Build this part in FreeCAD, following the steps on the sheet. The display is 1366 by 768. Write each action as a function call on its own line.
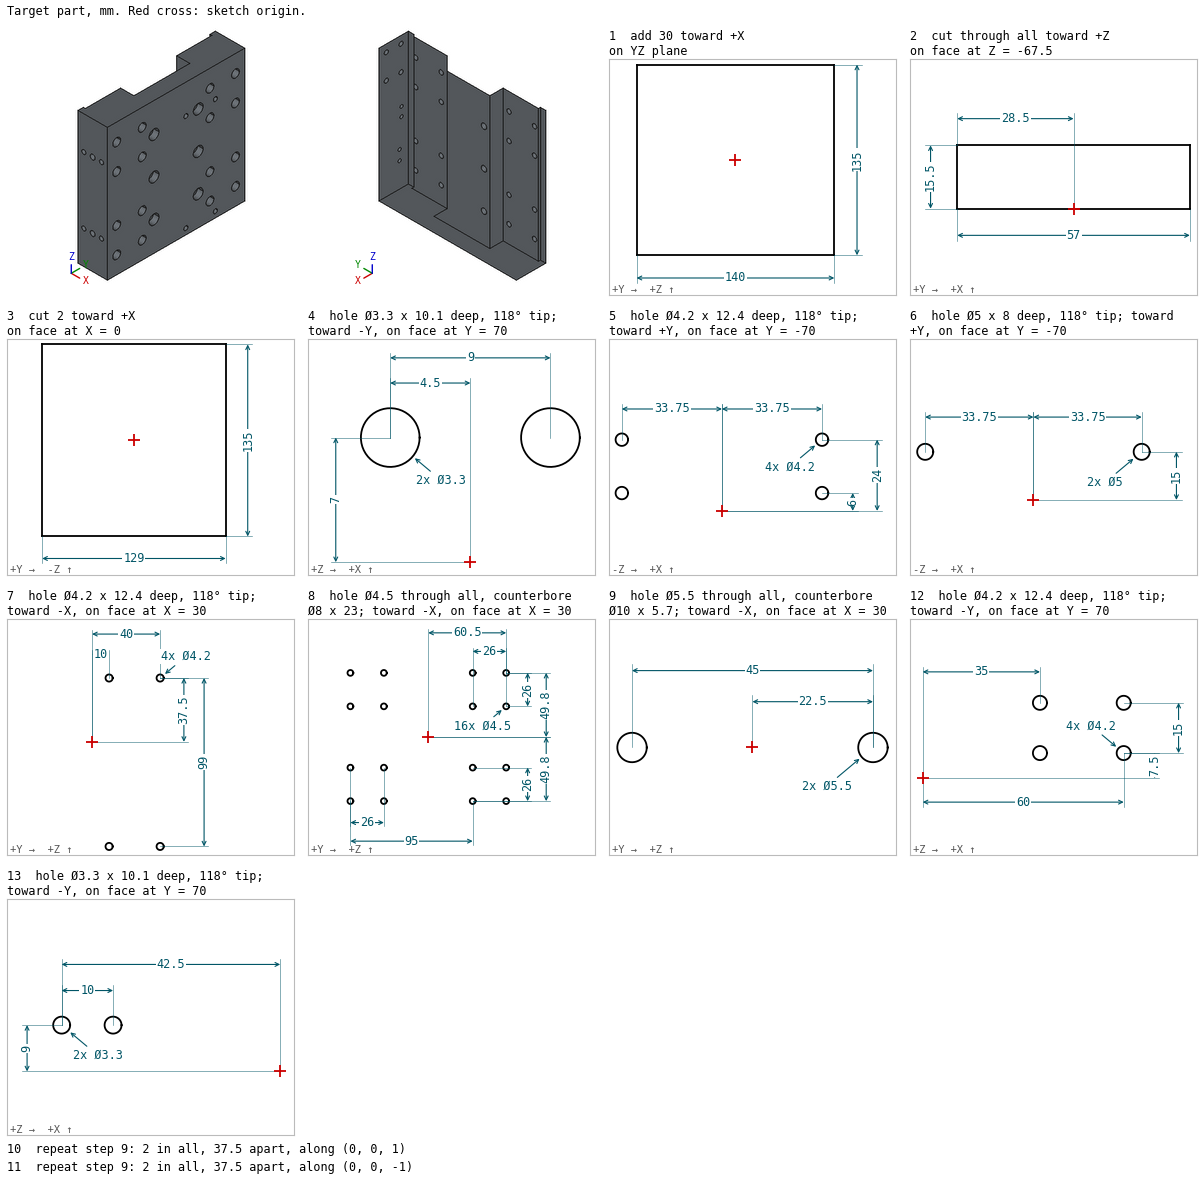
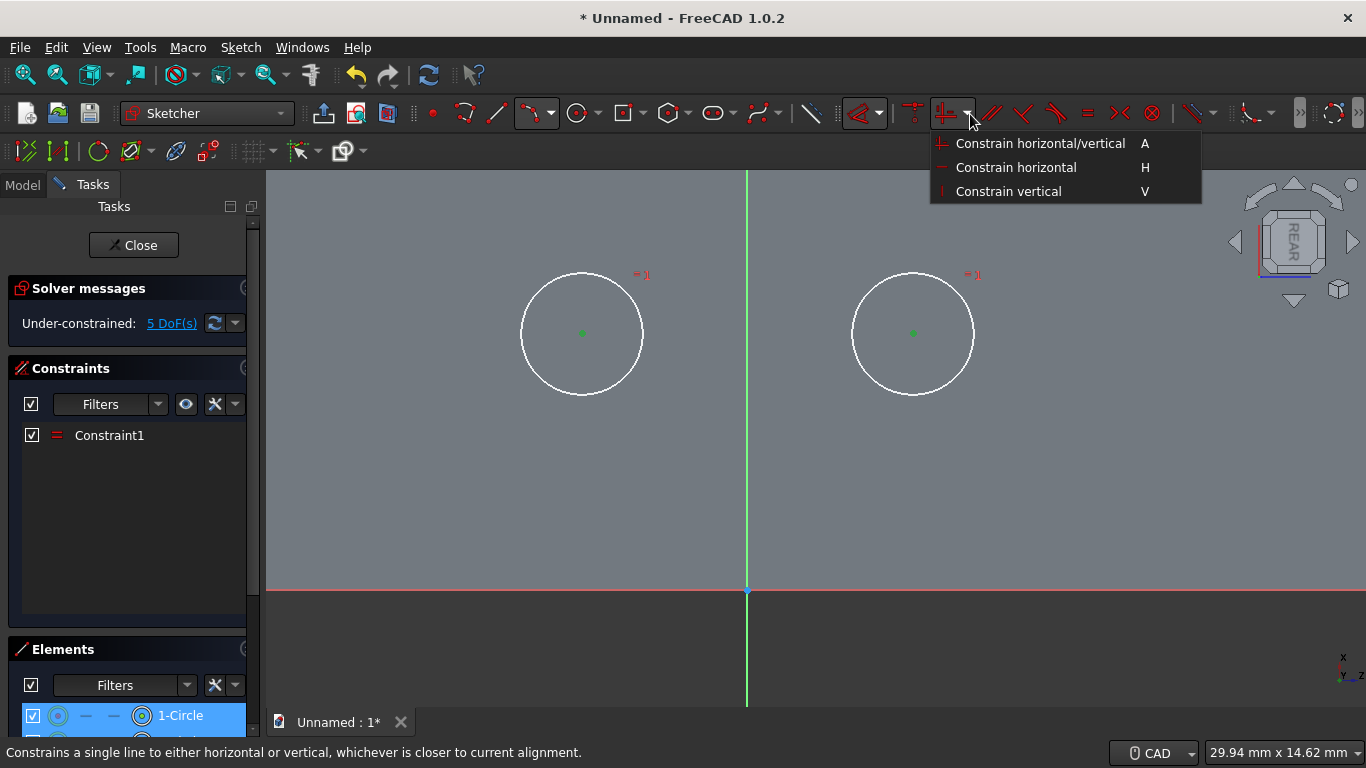
click(1066, 167)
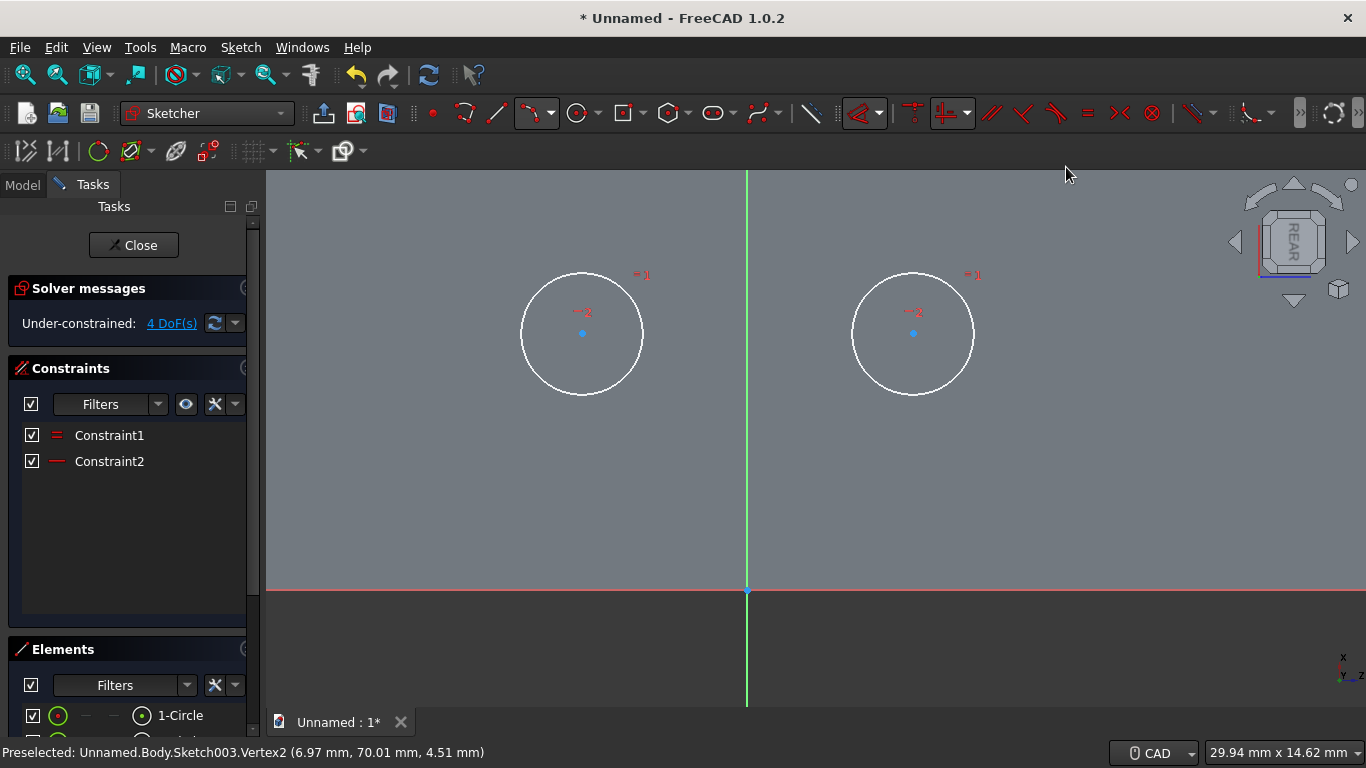
click(625, 291)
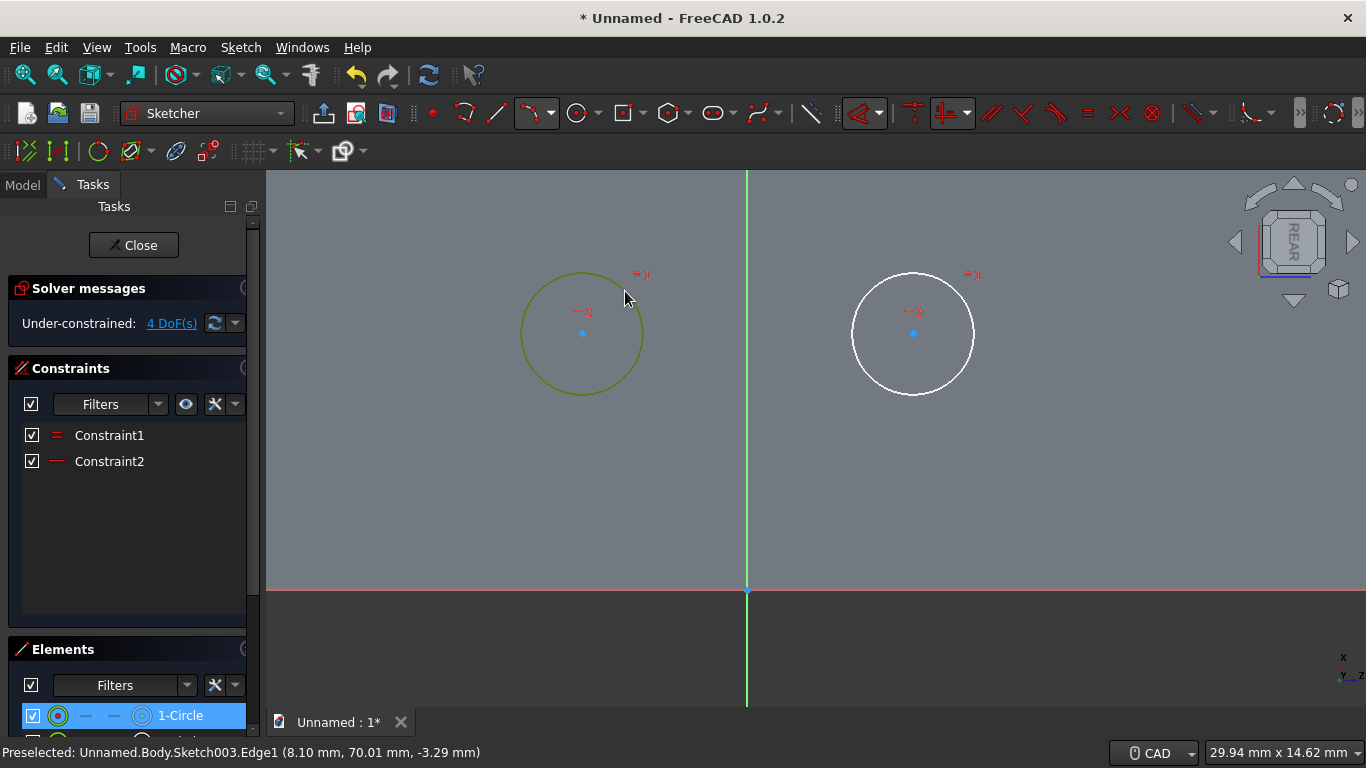
click(882, 114)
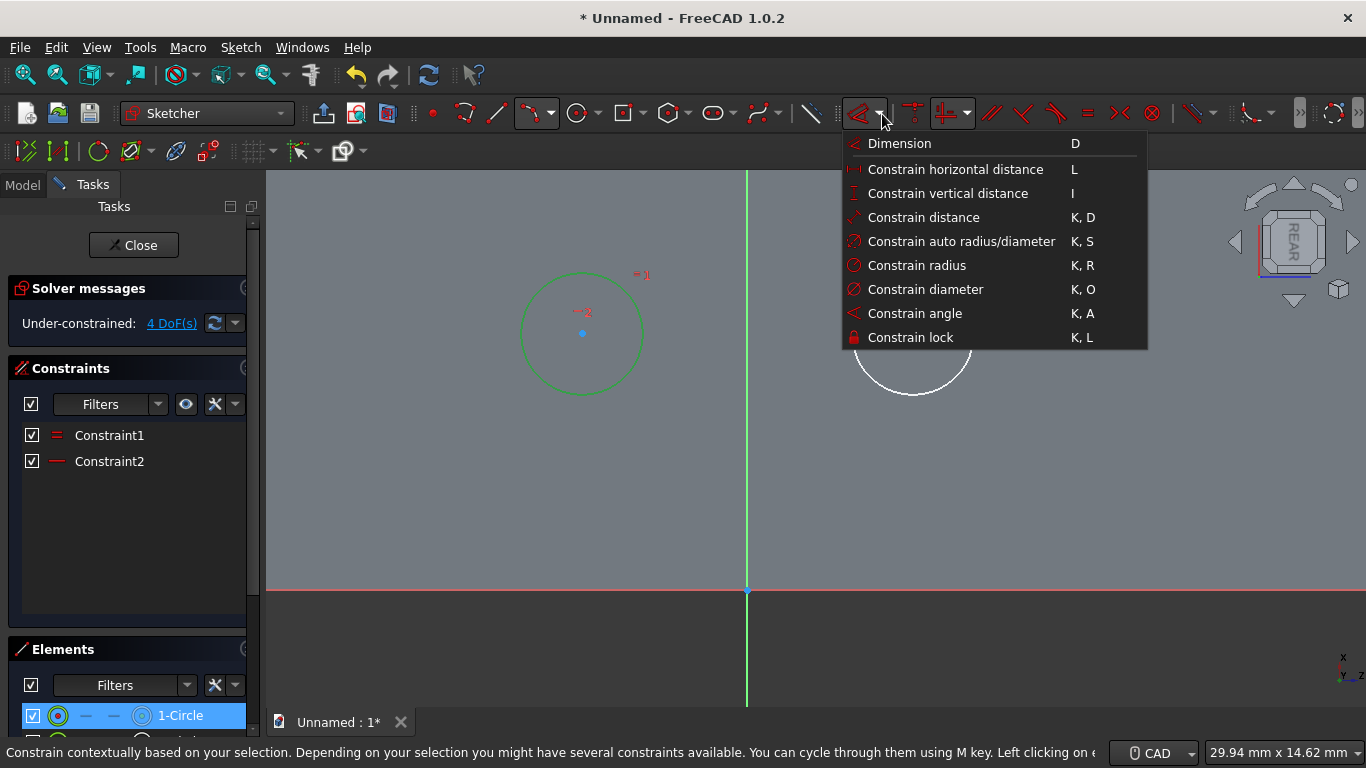
click(995, 289)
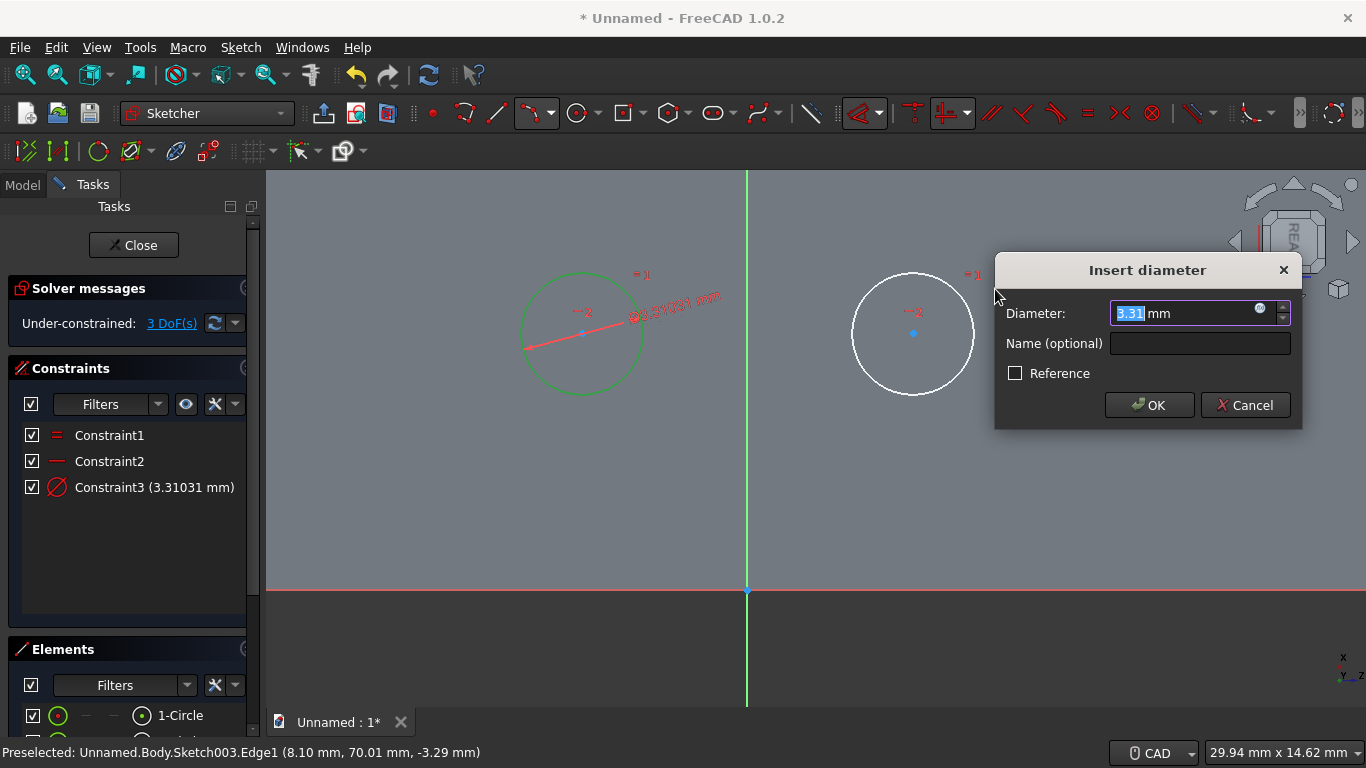
text(3.3)
key(Return)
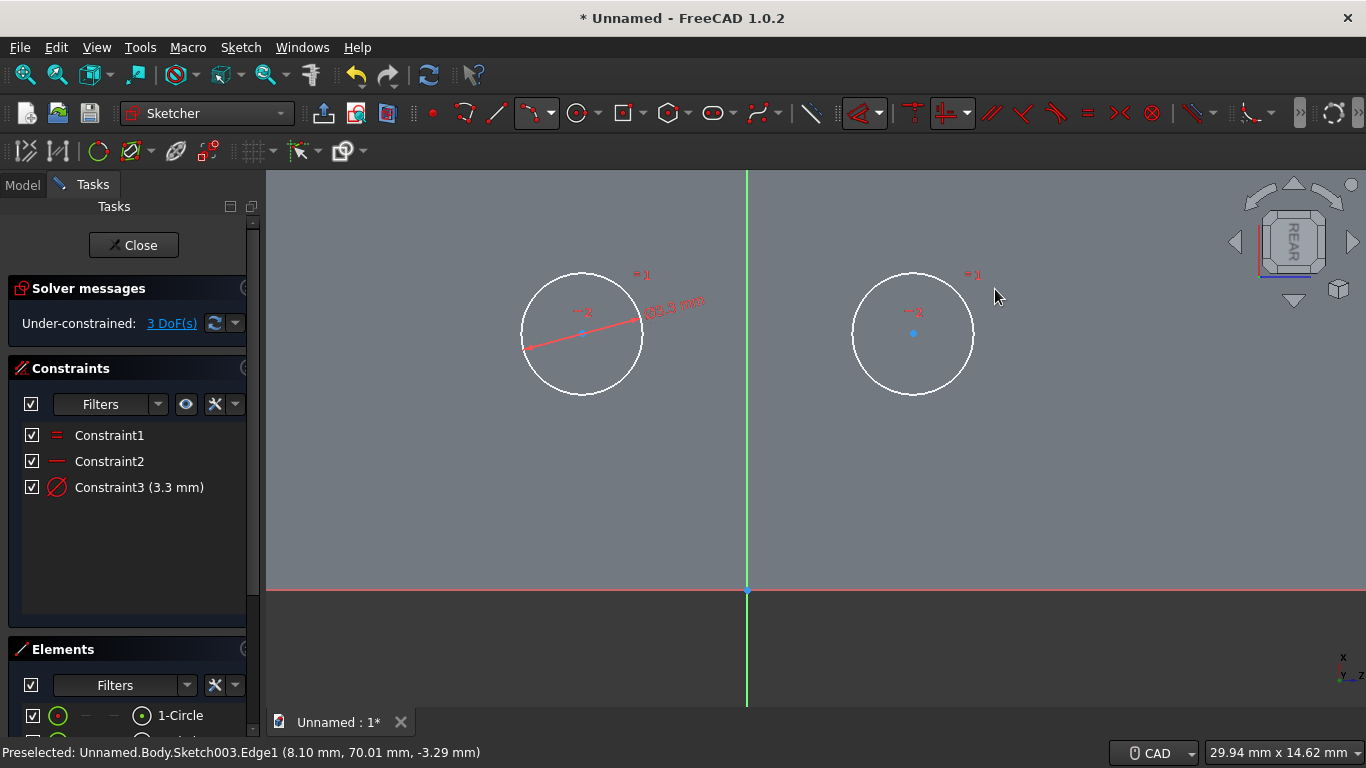
click(582, 334)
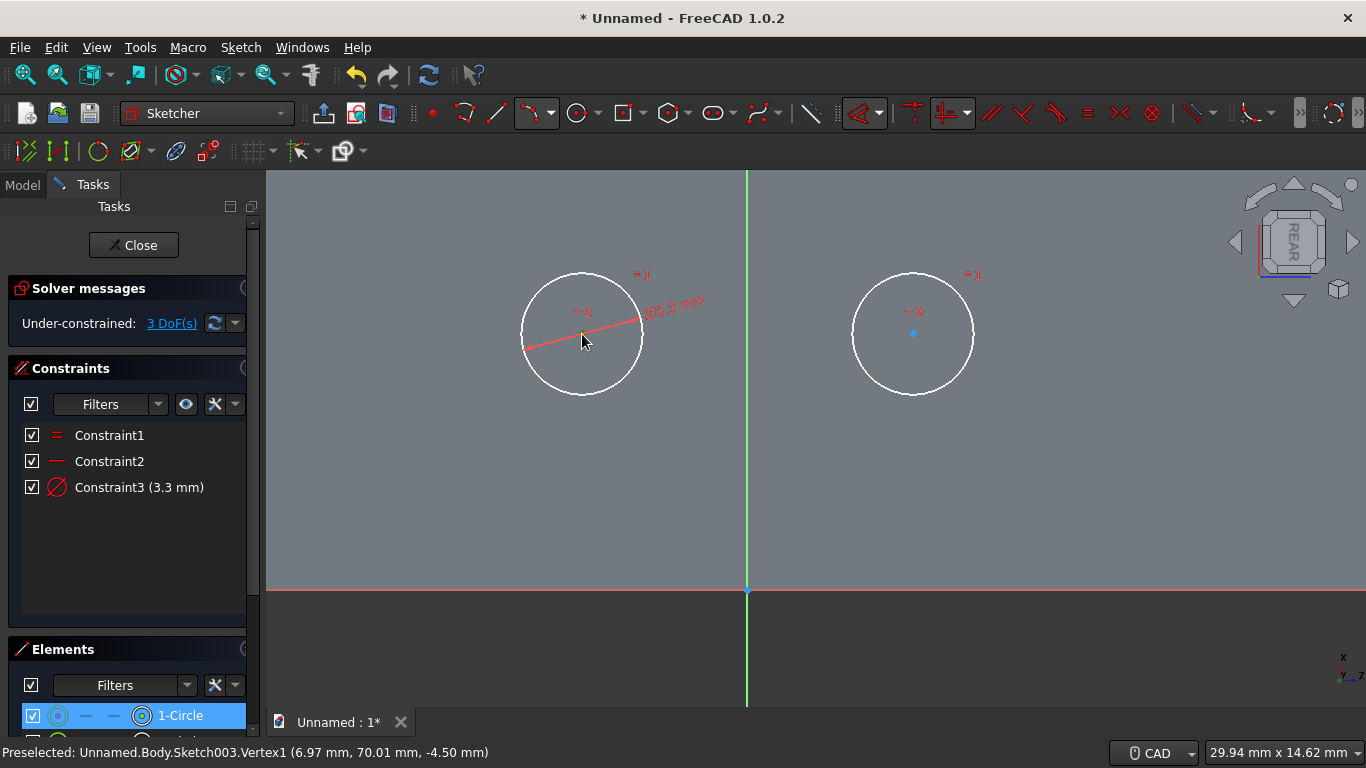
key(i)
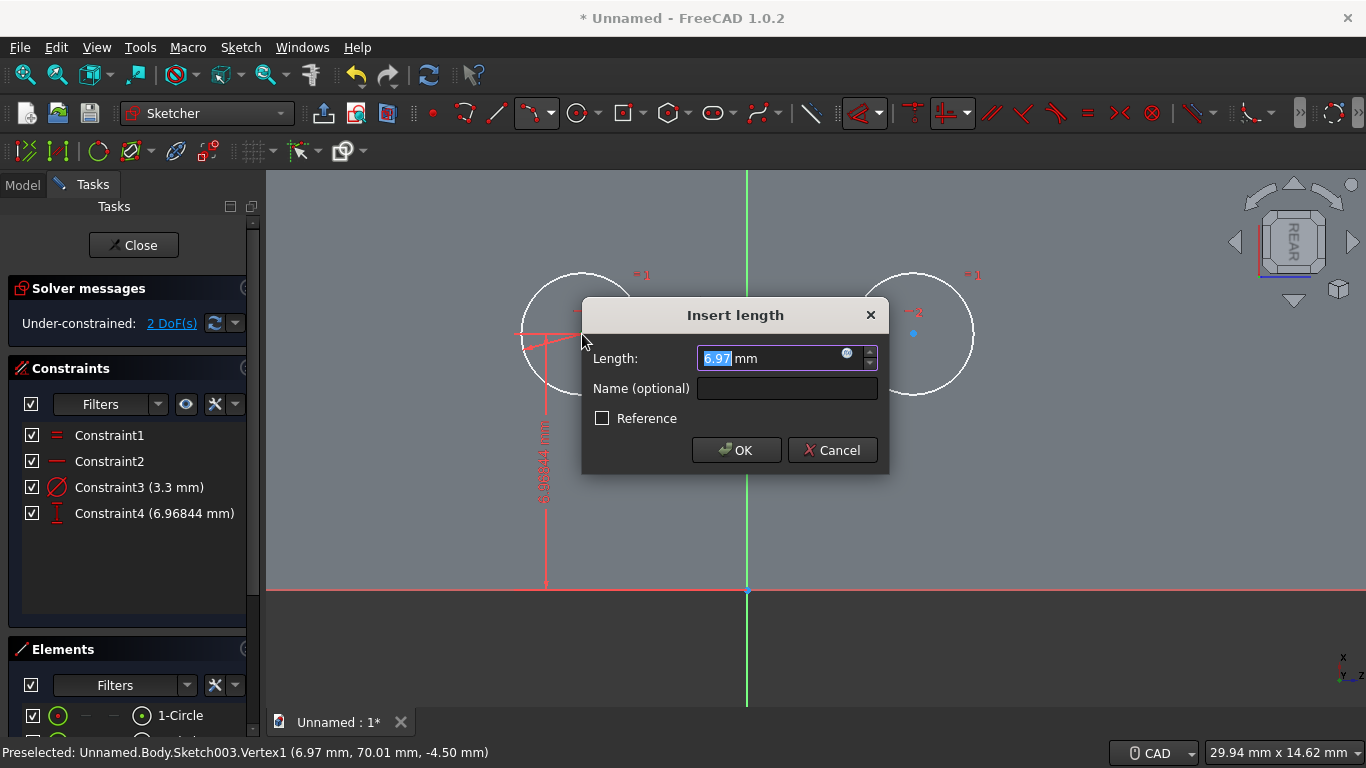
text(7)
key(Return)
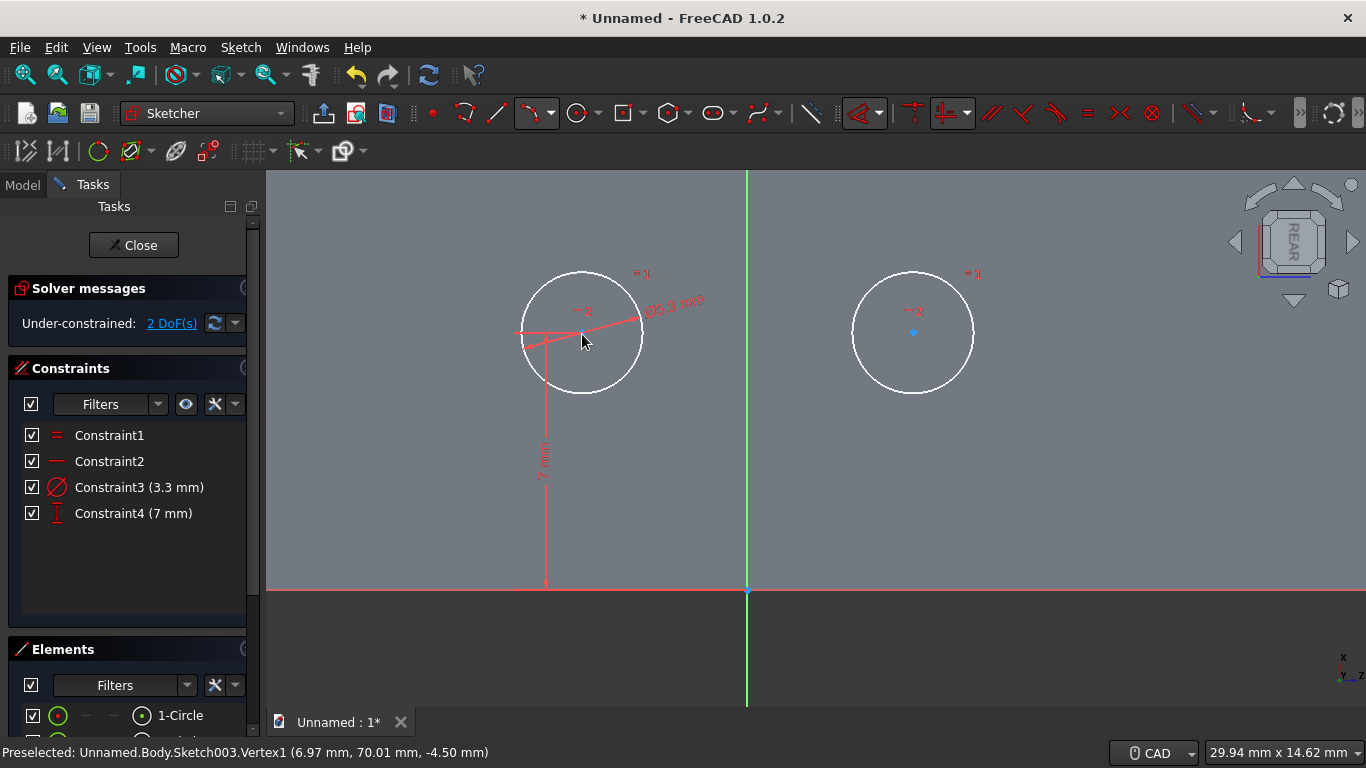
click(582, 333)